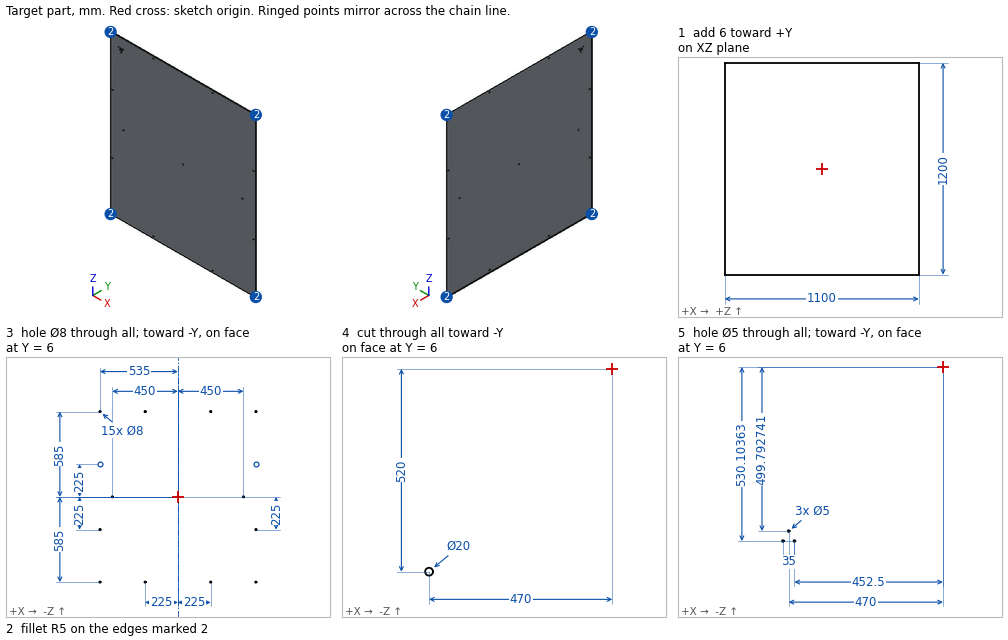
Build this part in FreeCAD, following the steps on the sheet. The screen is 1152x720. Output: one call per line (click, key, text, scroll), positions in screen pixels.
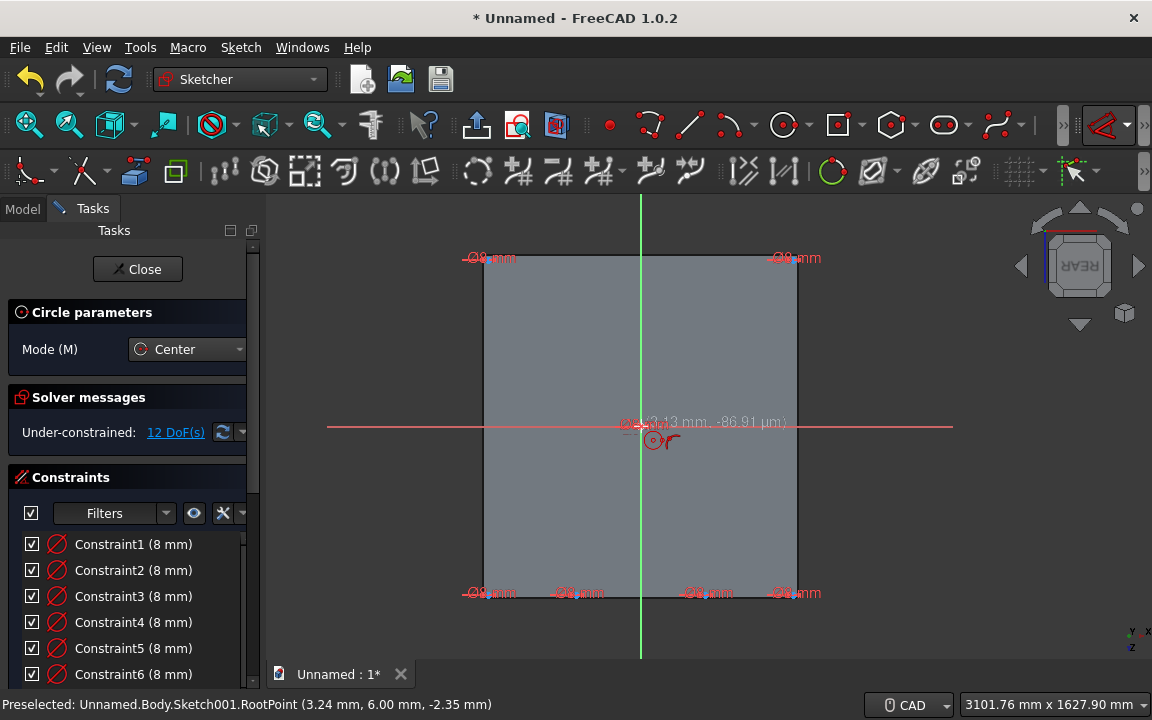
scroll(576, 259, up, 15)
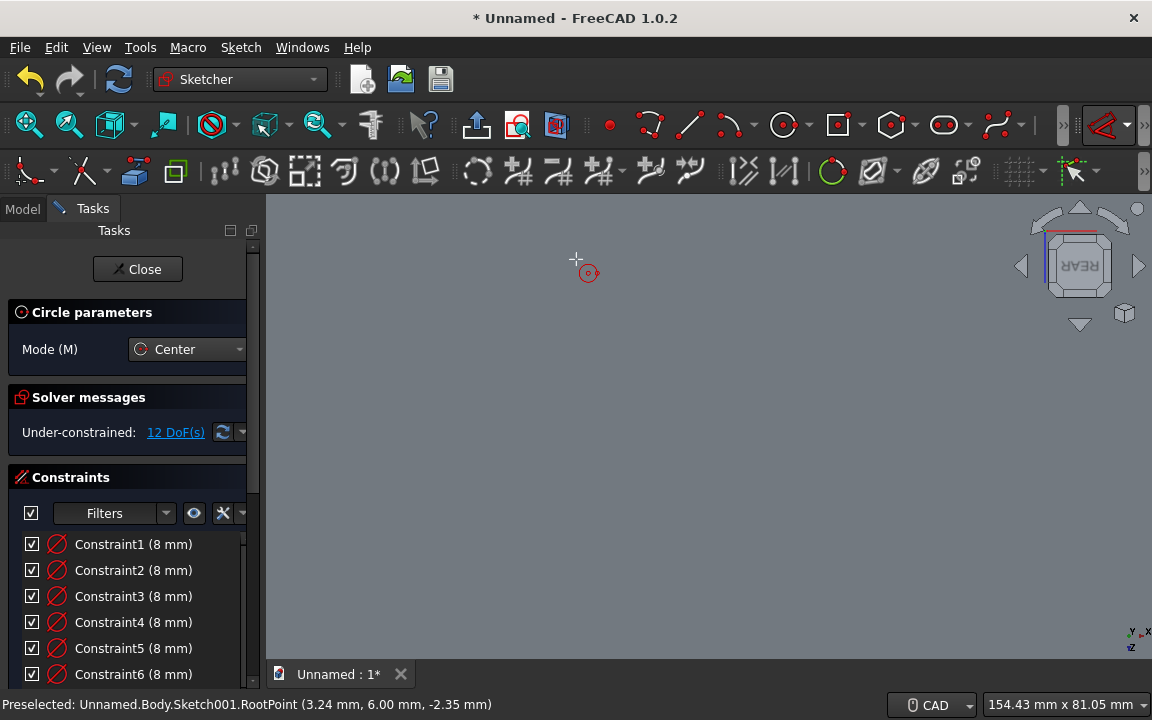
scroll(576, 259, down, 15)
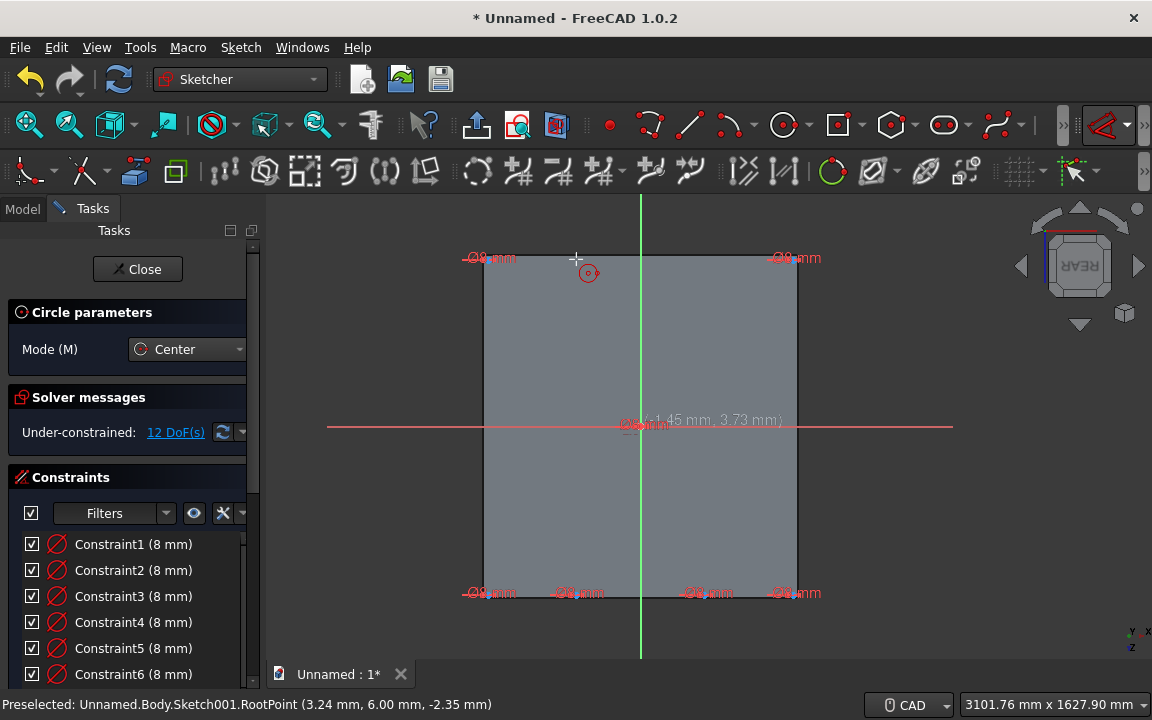
click(576, 259)
move(577, 259)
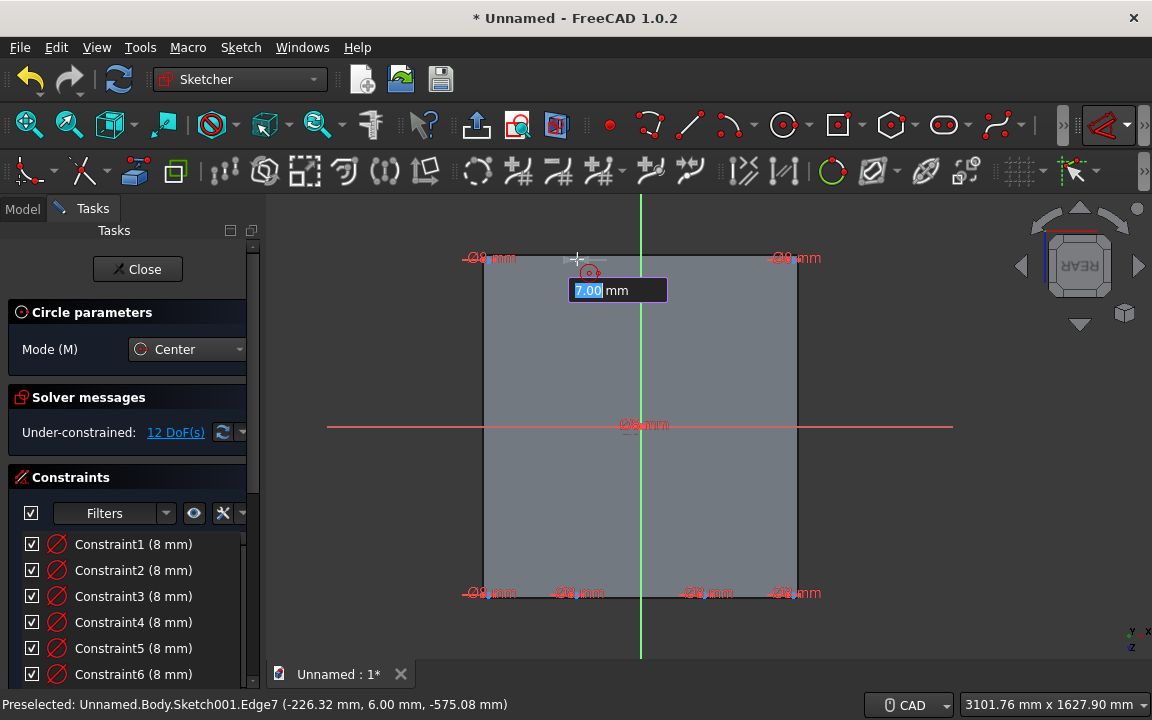
text(8)
key(Return)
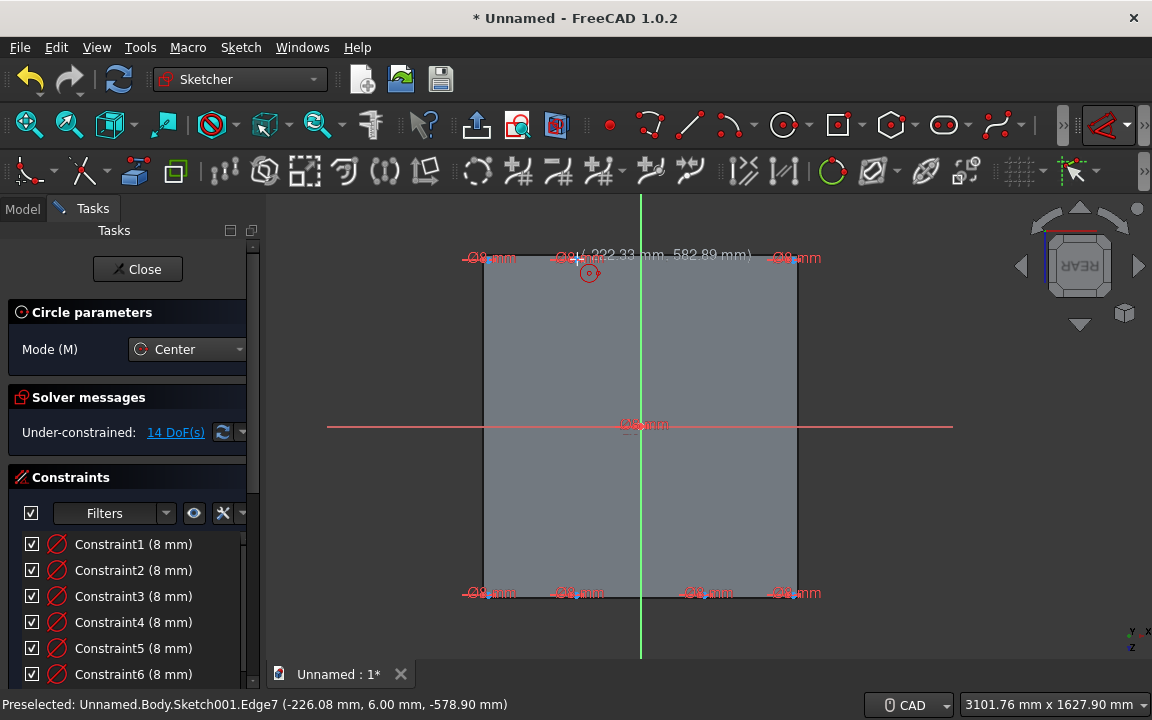
scroll(705, 259, up, 15)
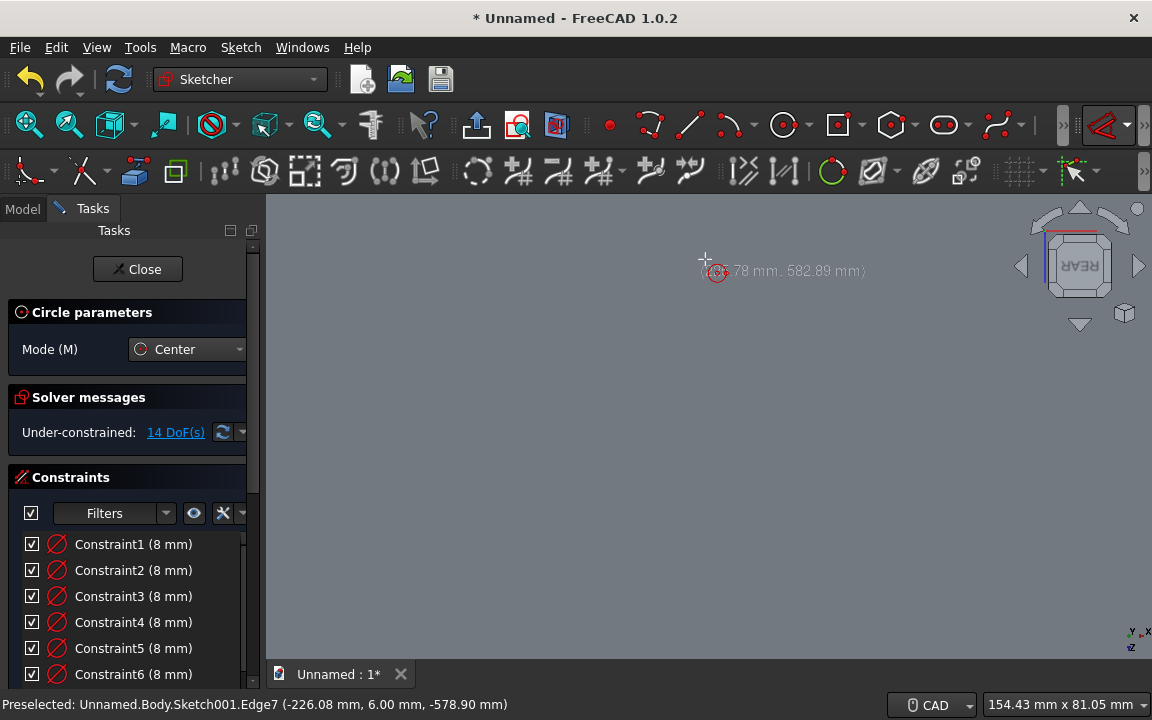
scroll(705, 259, down, 15)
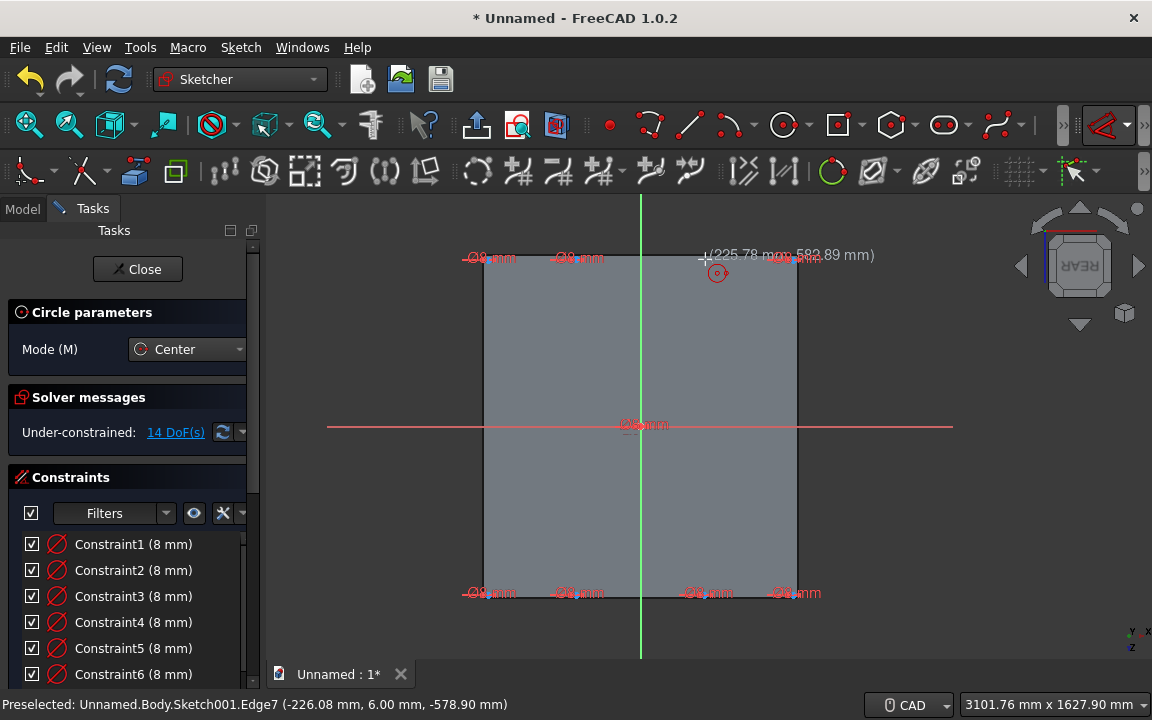
click(705, 259)
move(706, 259)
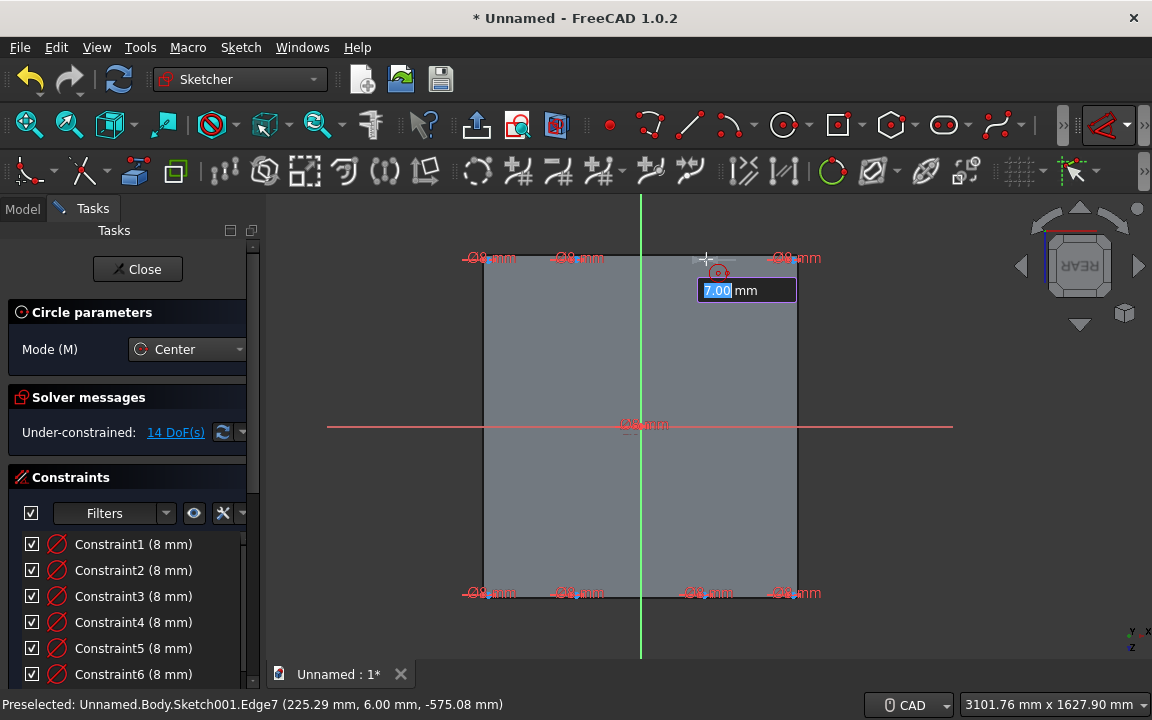
text(8)
key(Return)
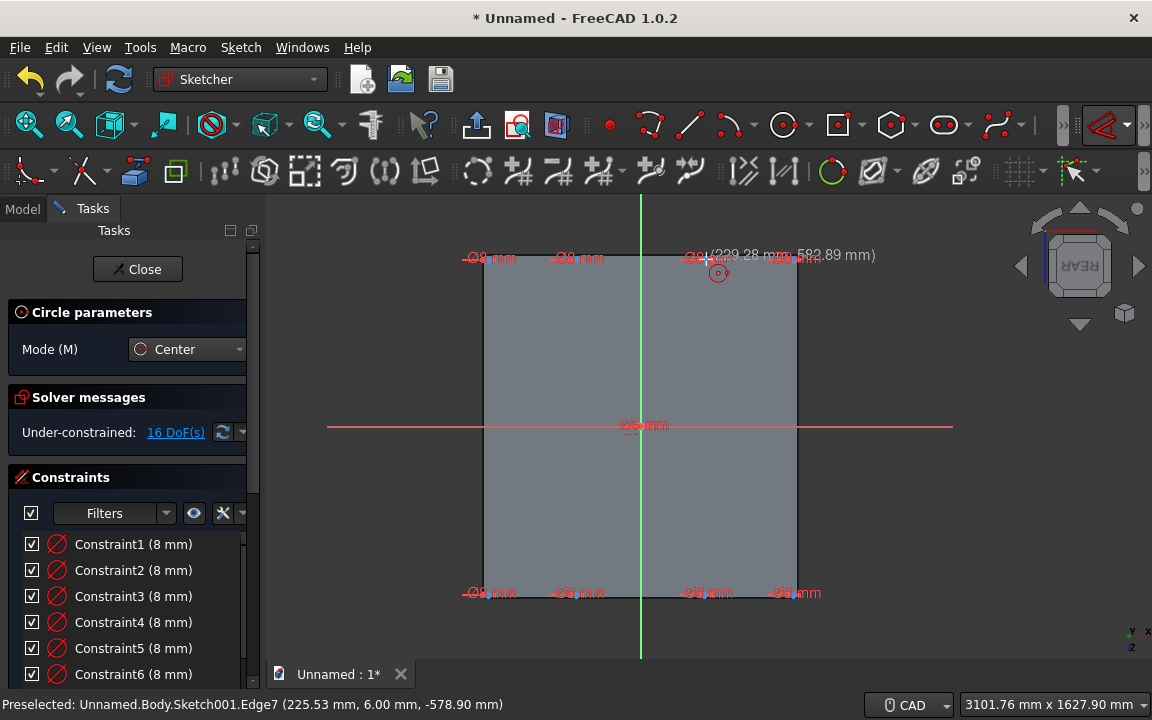
scroll(488, 491, up, 15)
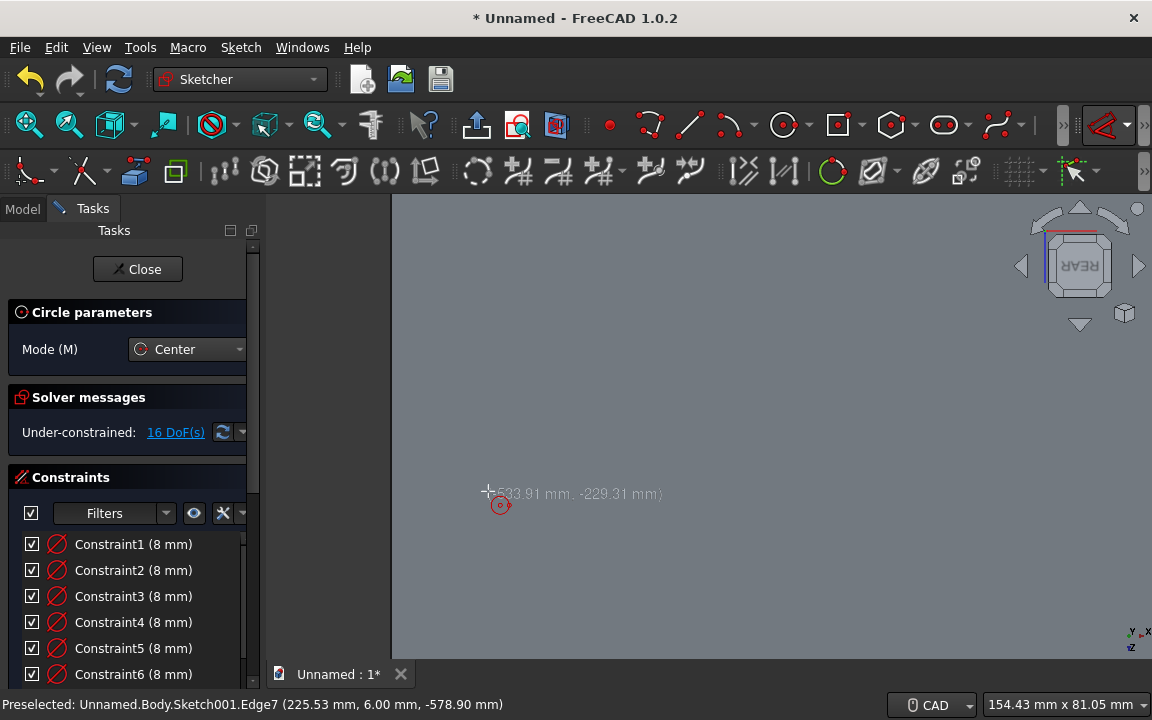
scroll(488, 492, down, 15)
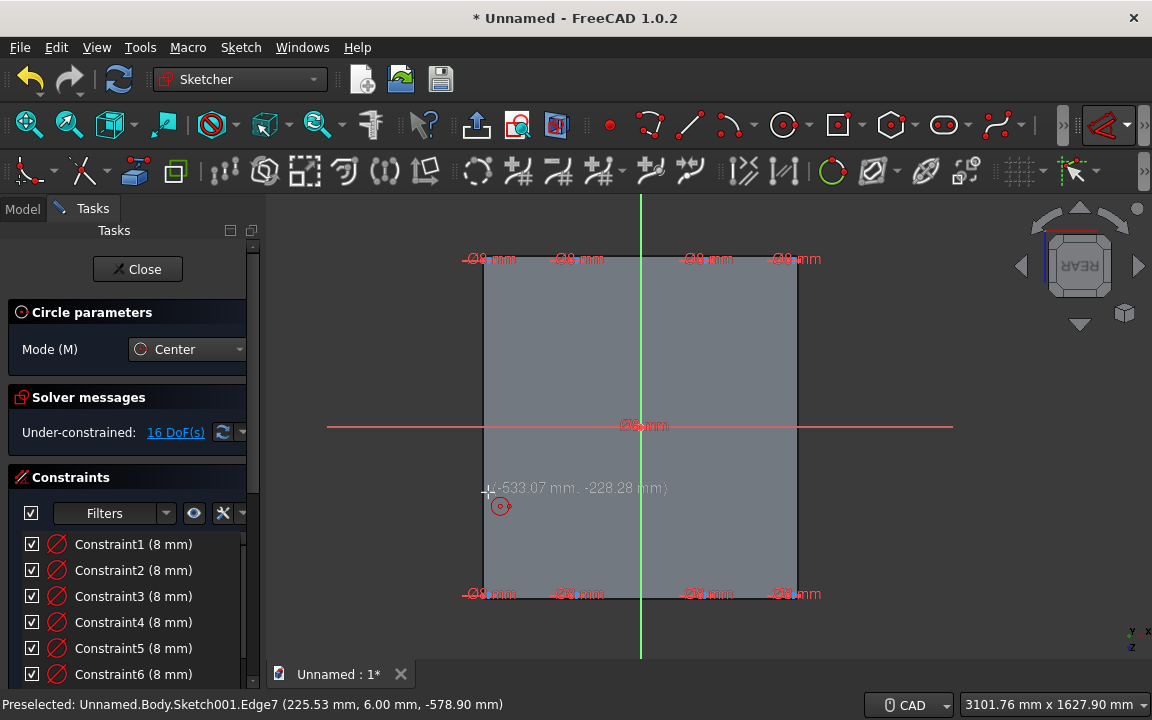
click(488, 492)
move(488, 491)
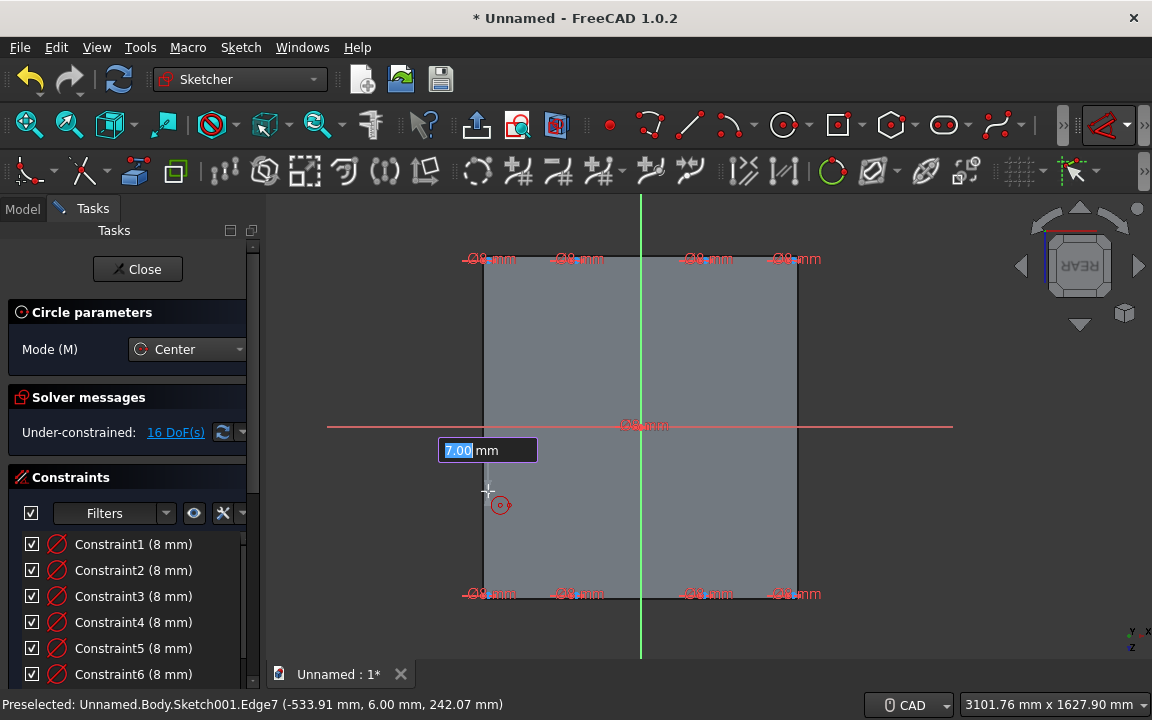
text(8)
key(Return)